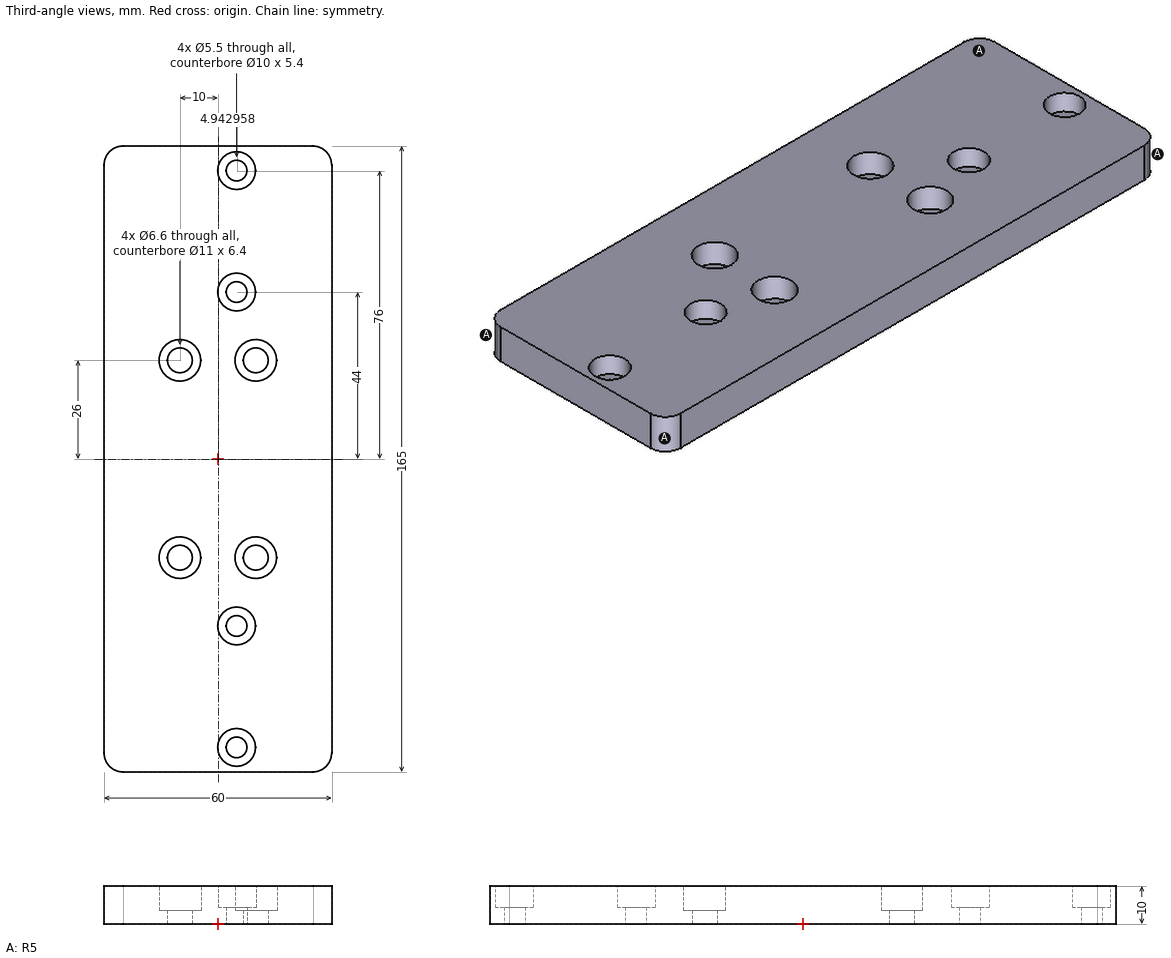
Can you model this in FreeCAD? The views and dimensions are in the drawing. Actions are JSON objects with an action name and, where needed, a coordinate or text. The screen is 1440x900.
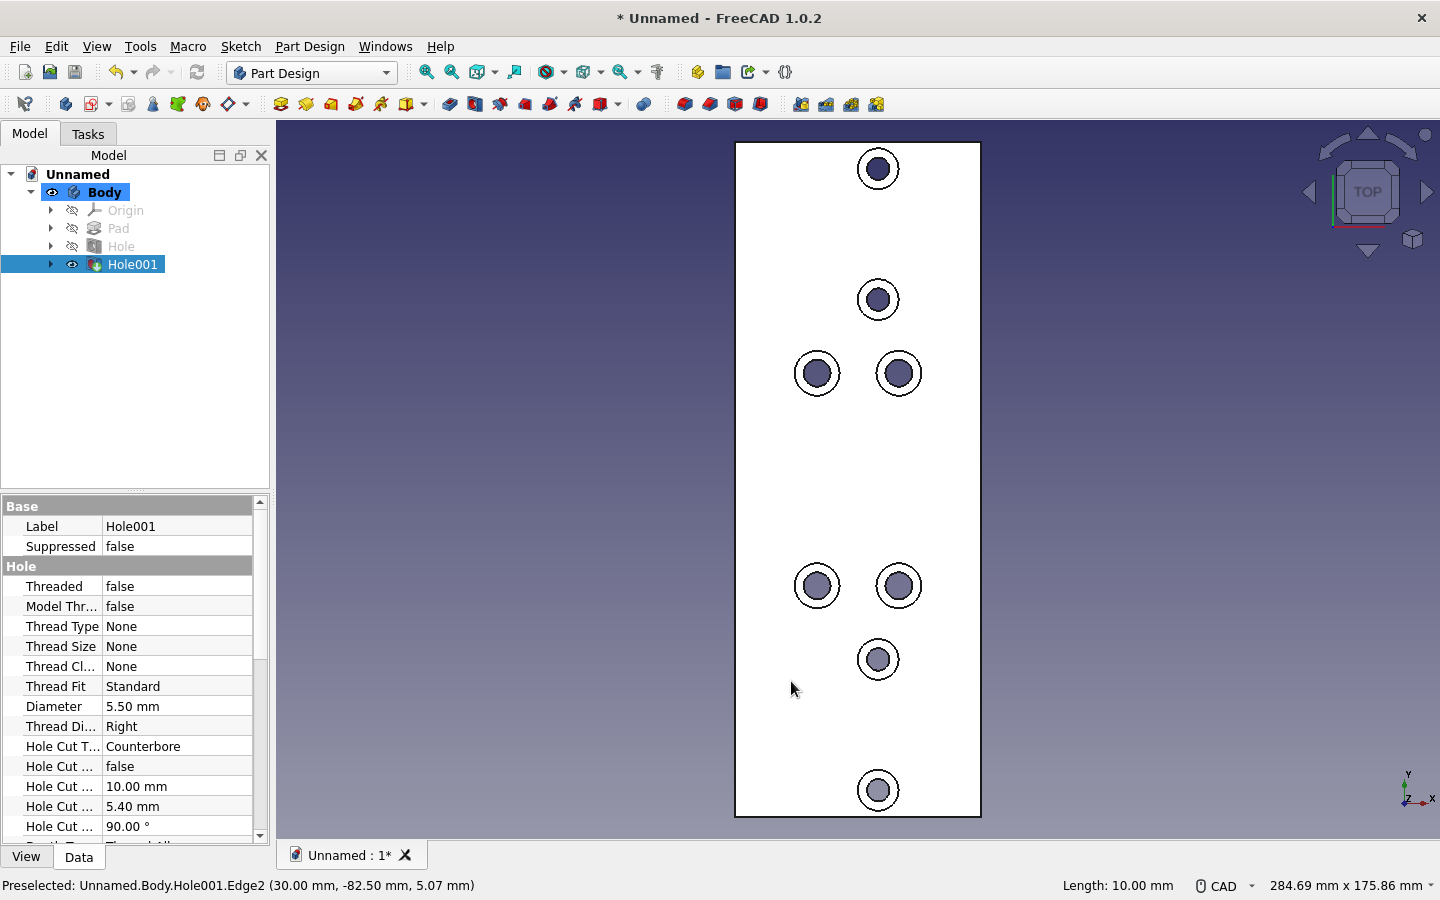
{"action": "key", "text": "1"}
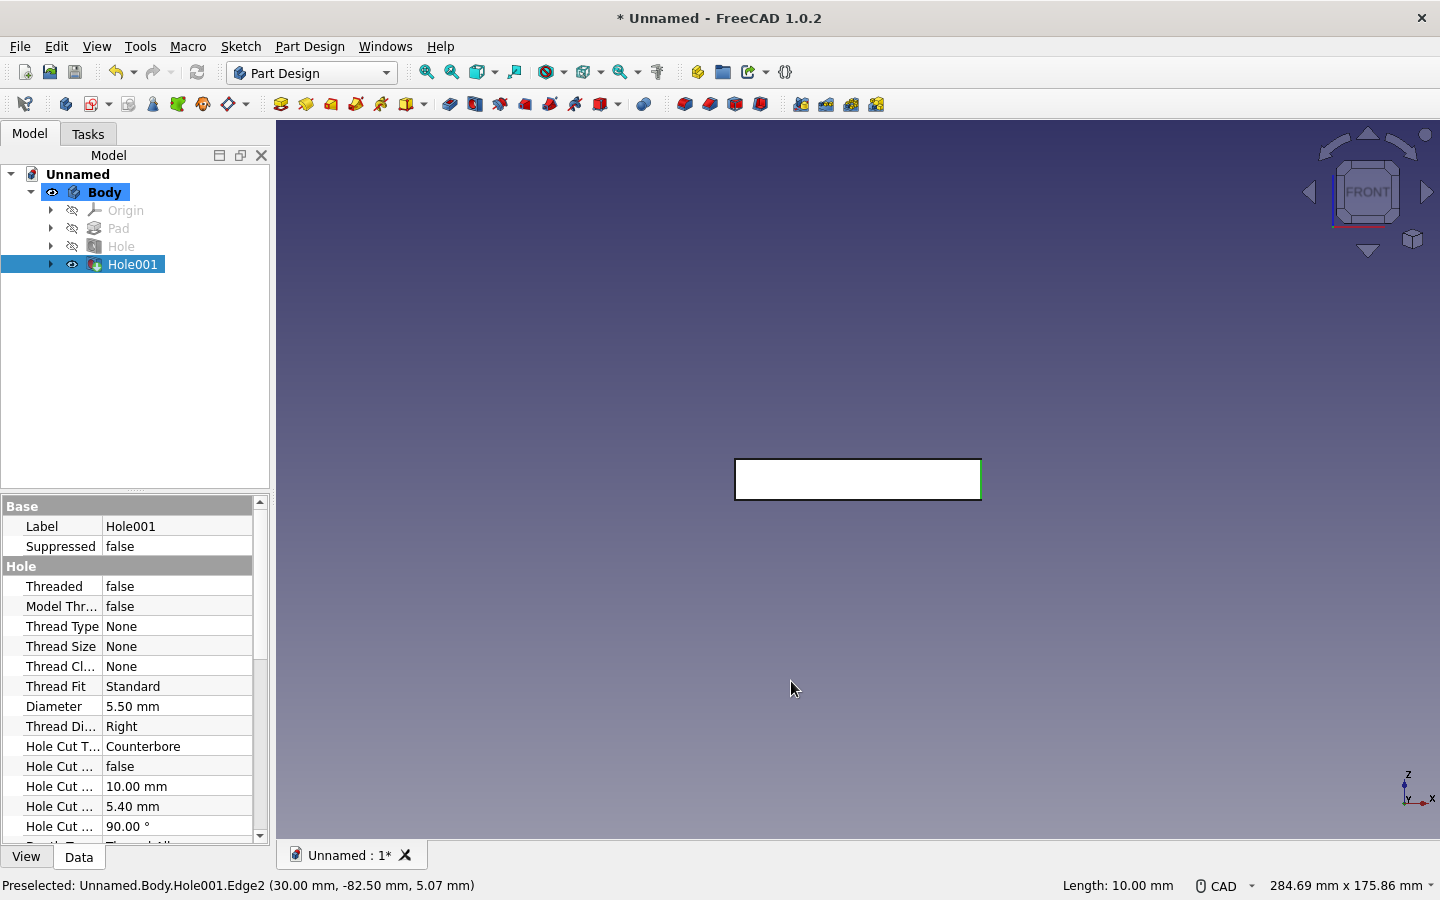
{"action": "key", "text": "v f"}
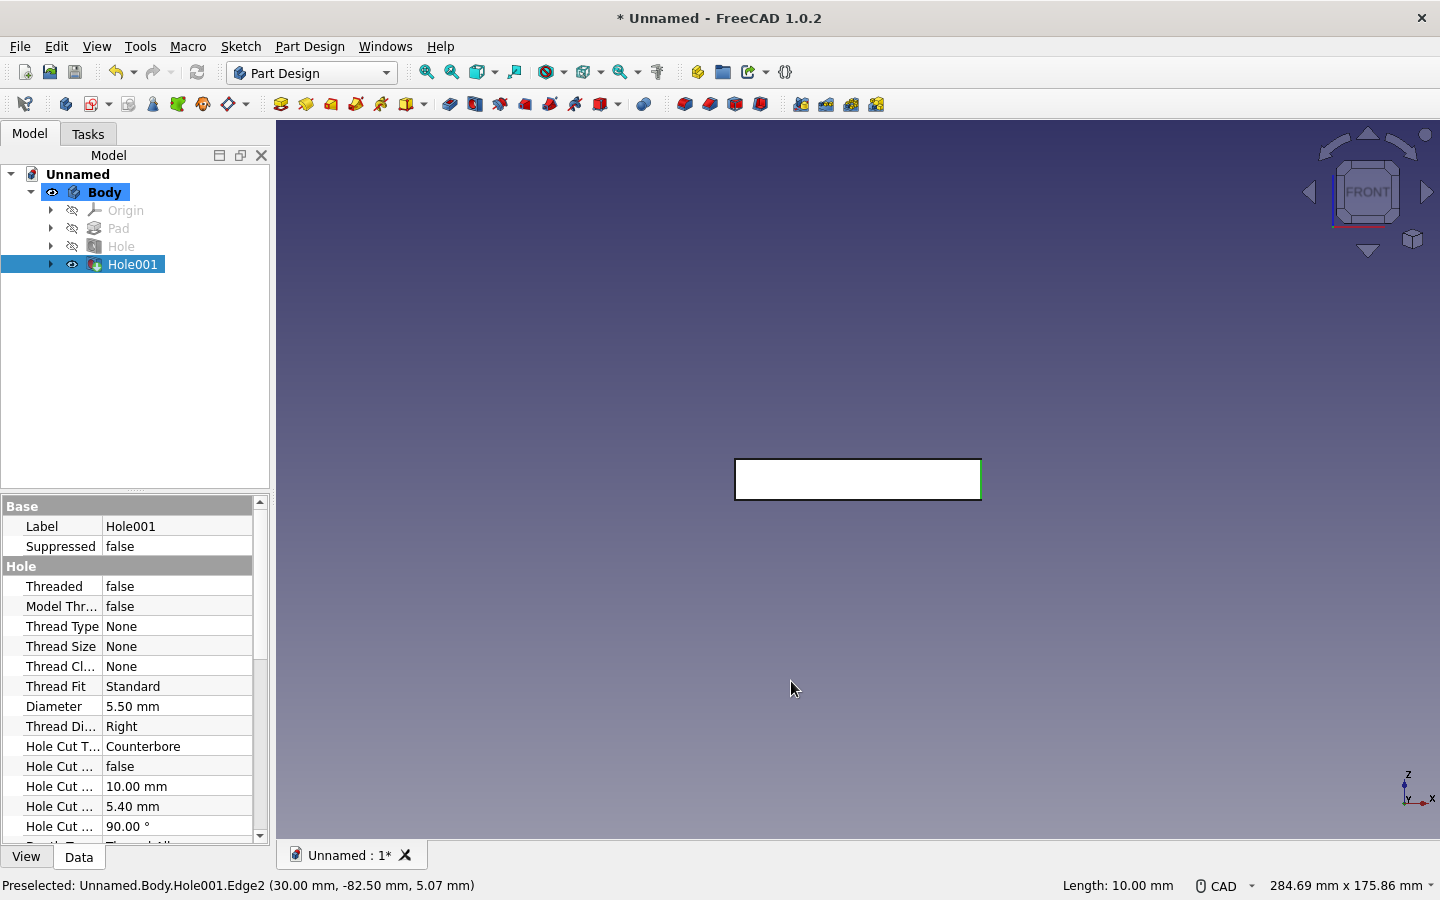
{"action": "left_click", "coordinate": [735, 479], "text": "ctrl"}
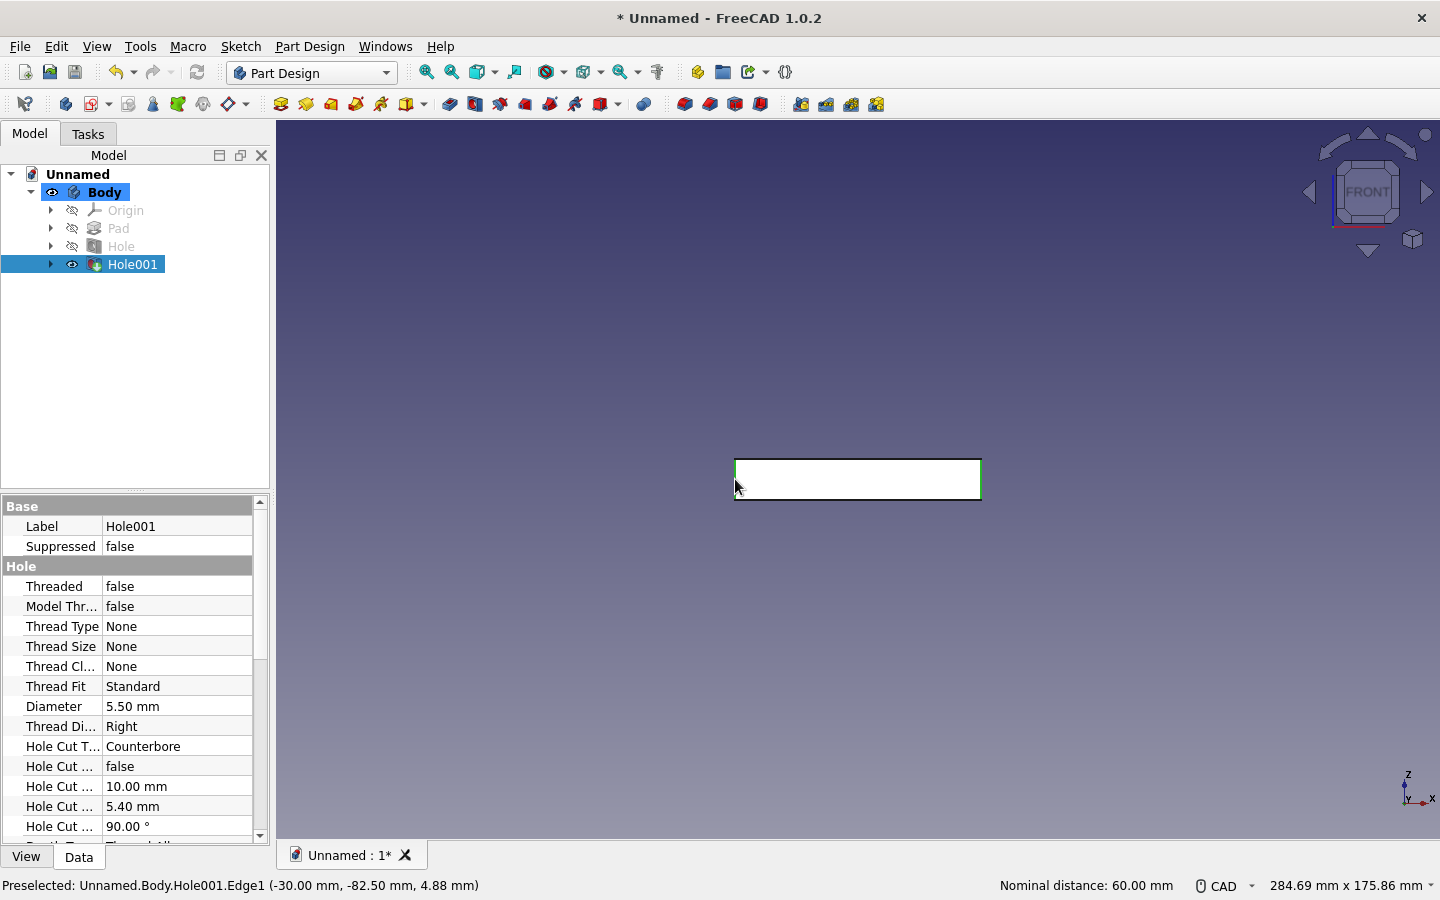
{"action": "key", "text": "3"}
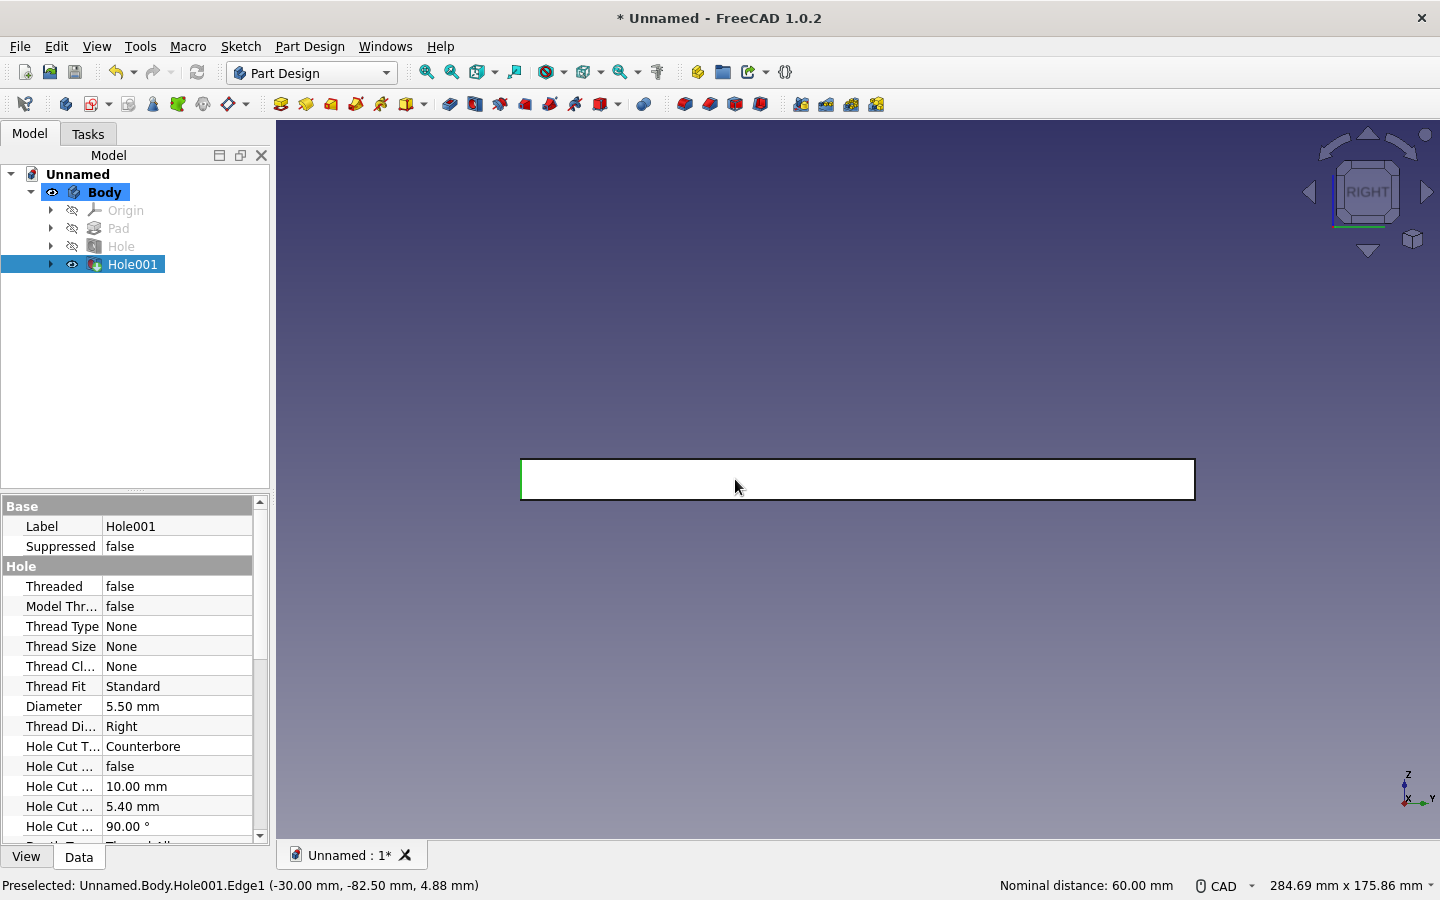
{"action": "left_click", "coordinate": [1195, 478], "text": "ctrl"}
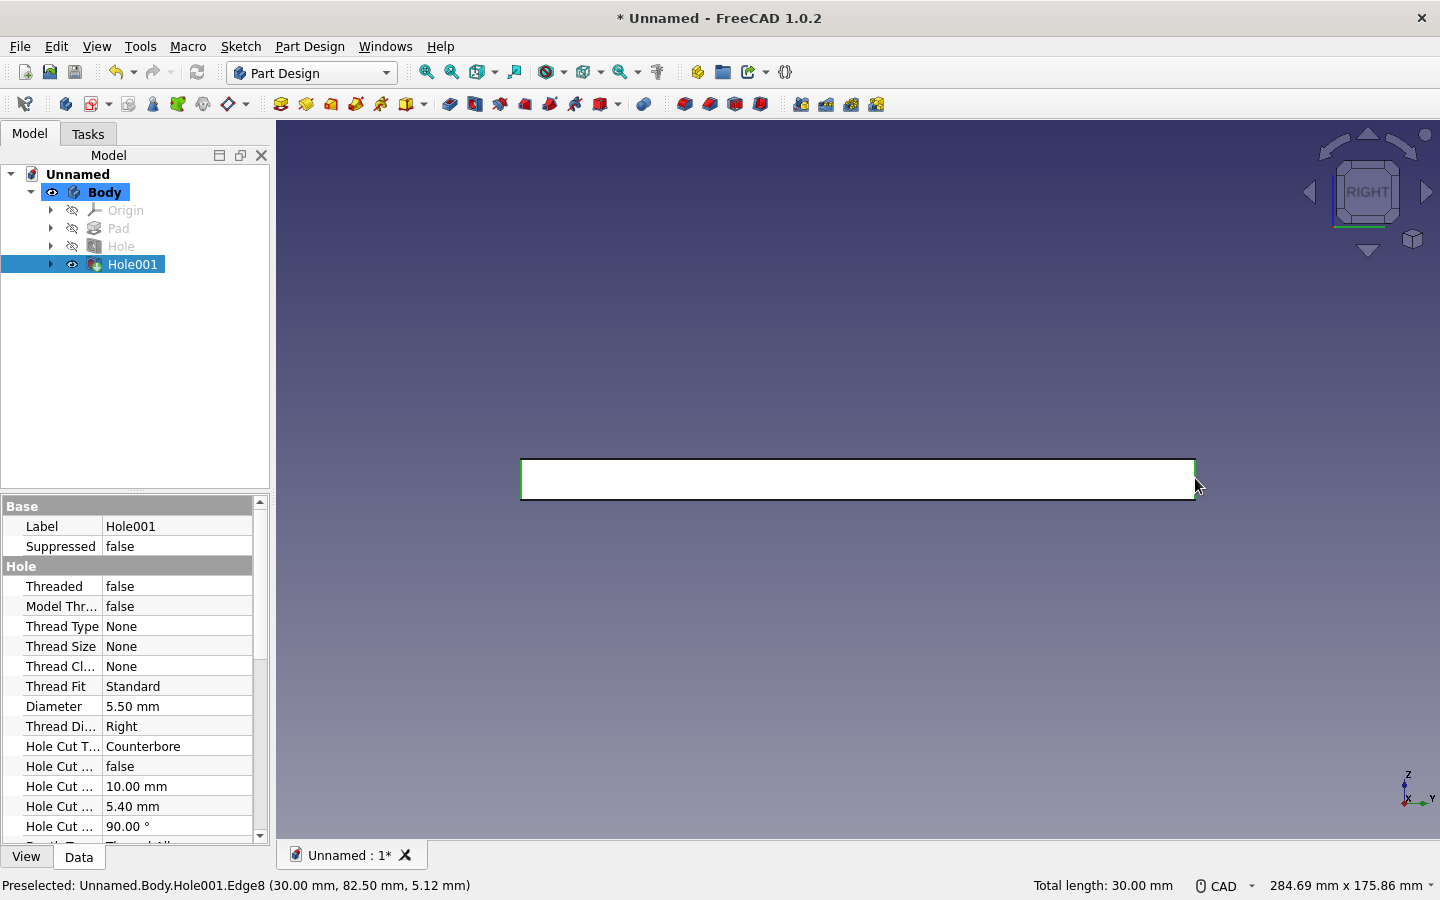
{"action": "key", "text": "5"}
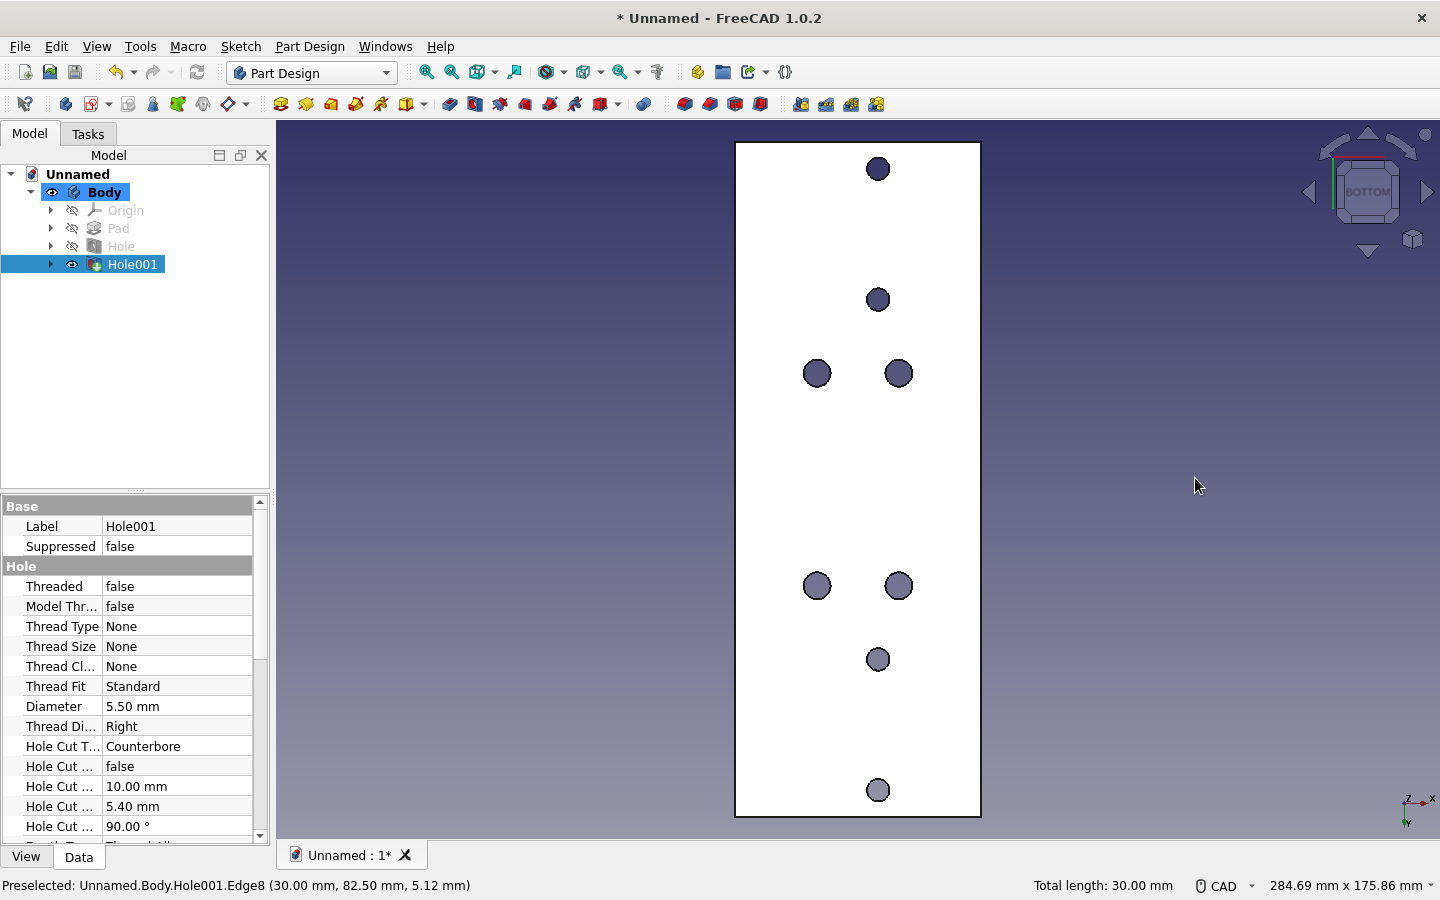
{"action": "key", "text": "4"}